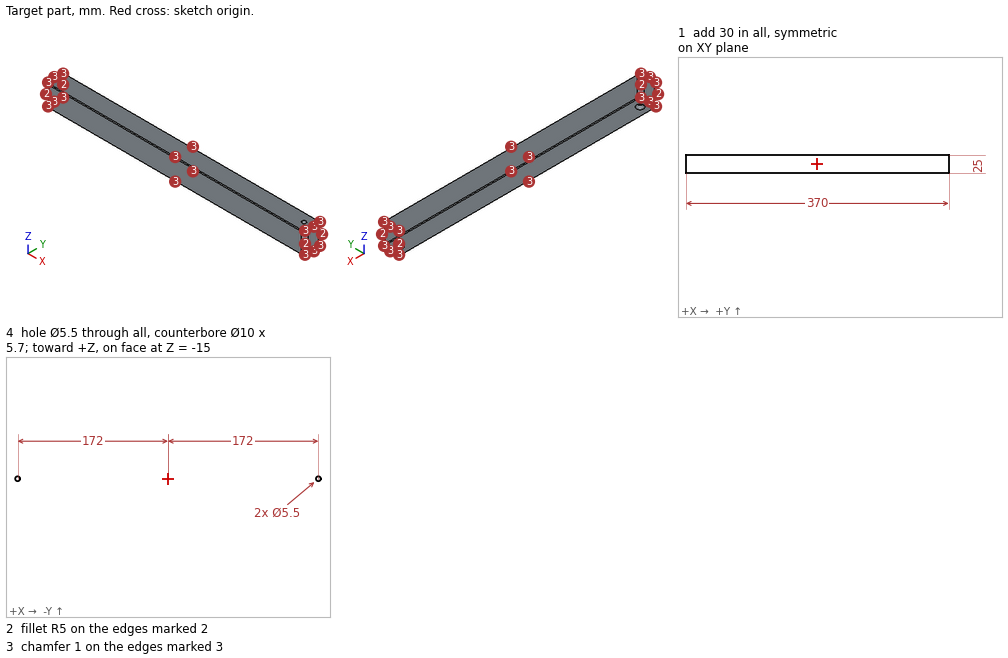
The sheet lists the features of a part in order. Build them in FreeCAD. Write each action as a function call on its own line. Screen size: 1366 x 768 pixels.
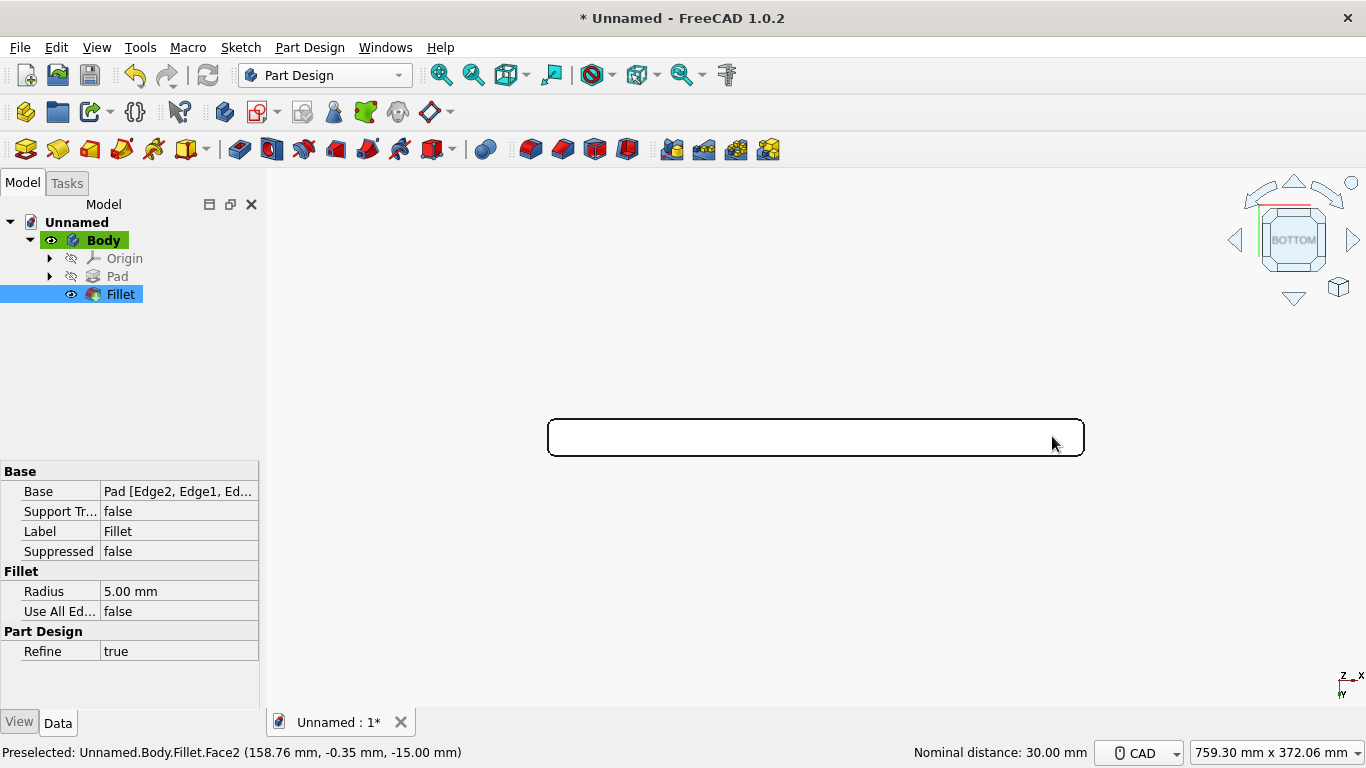
click(564, 150)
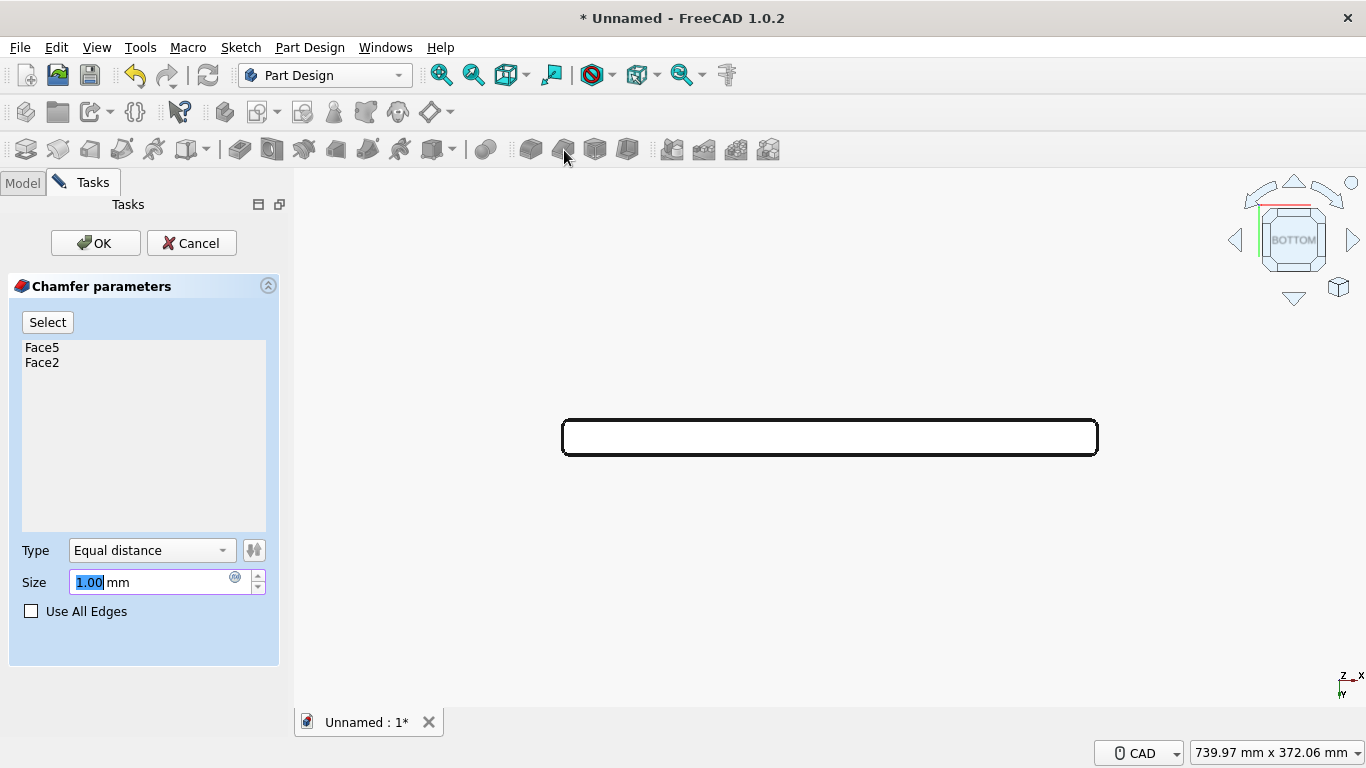
text(1)
key(Tab)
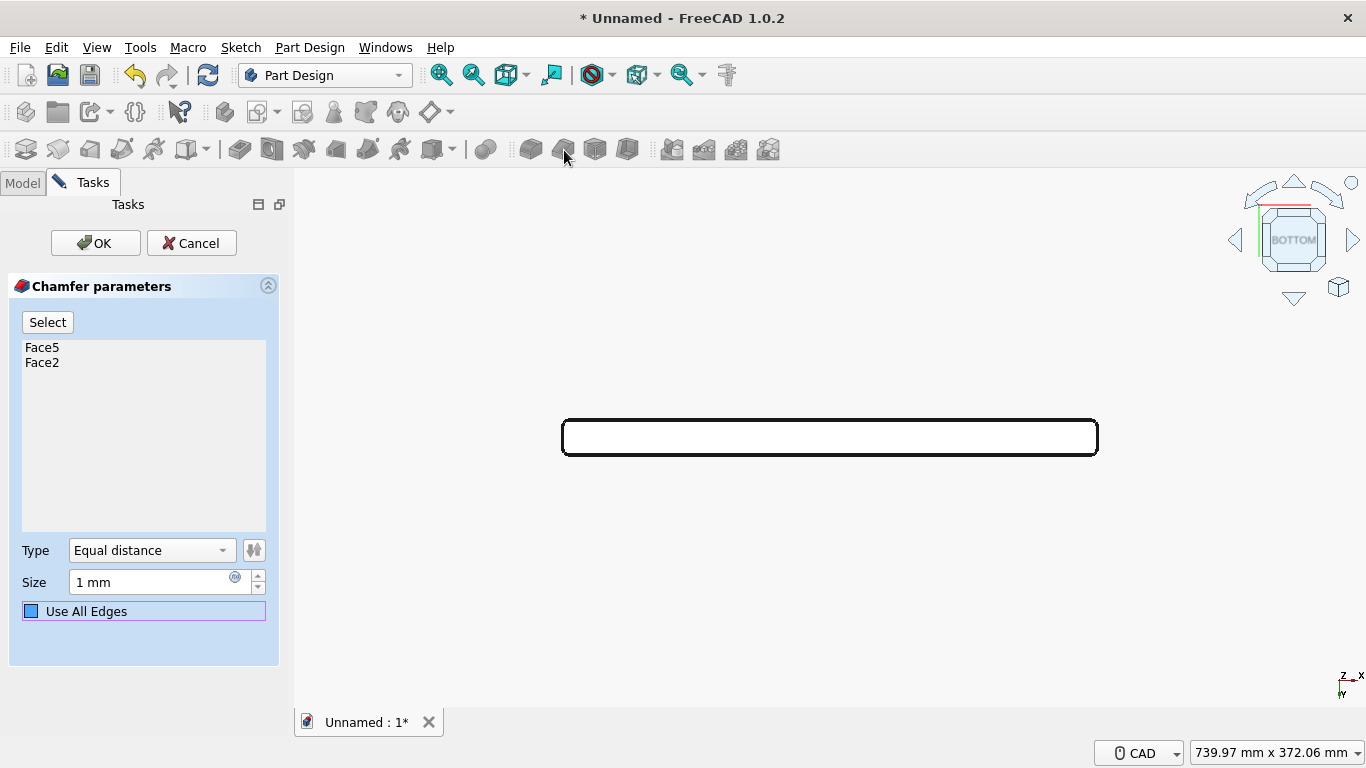
click(96, 243)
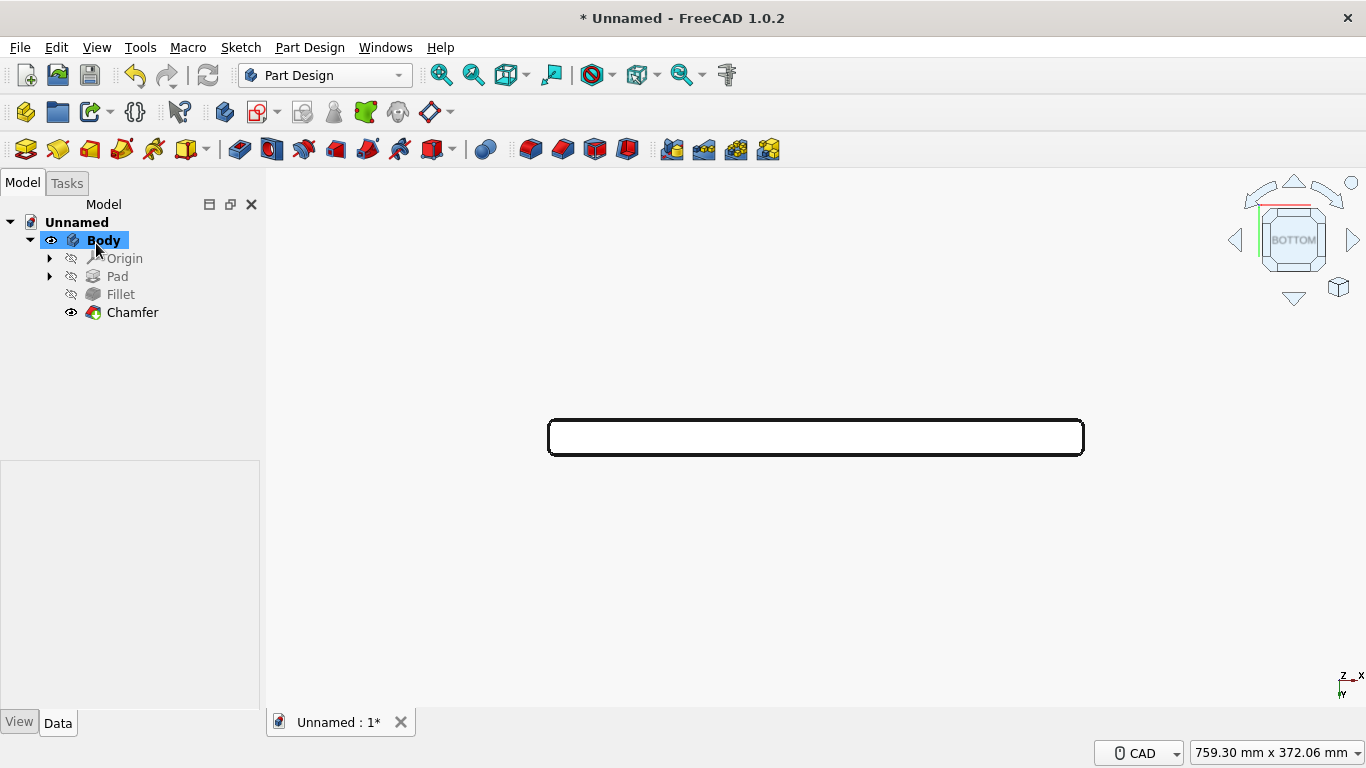
click(1044, 436)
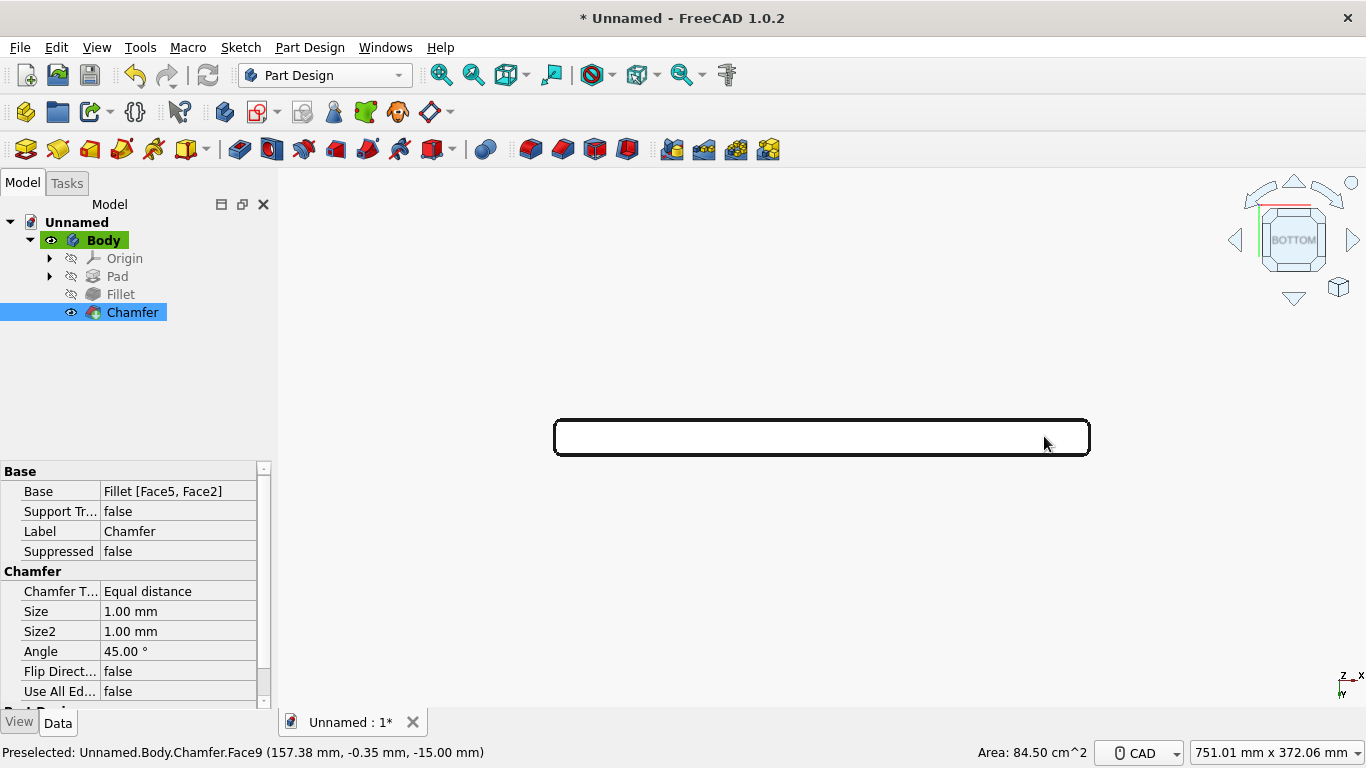
click(258, 112)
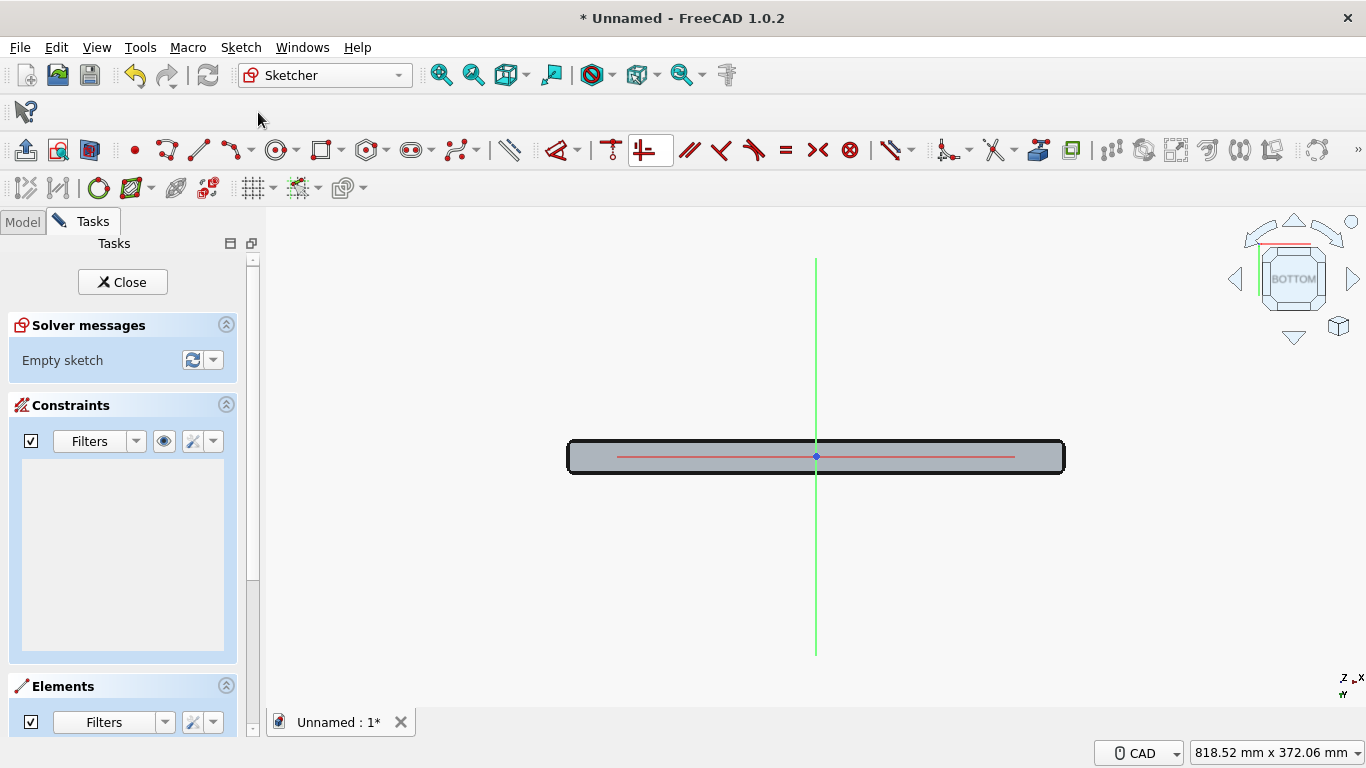
scroll(955, 457, up, 2)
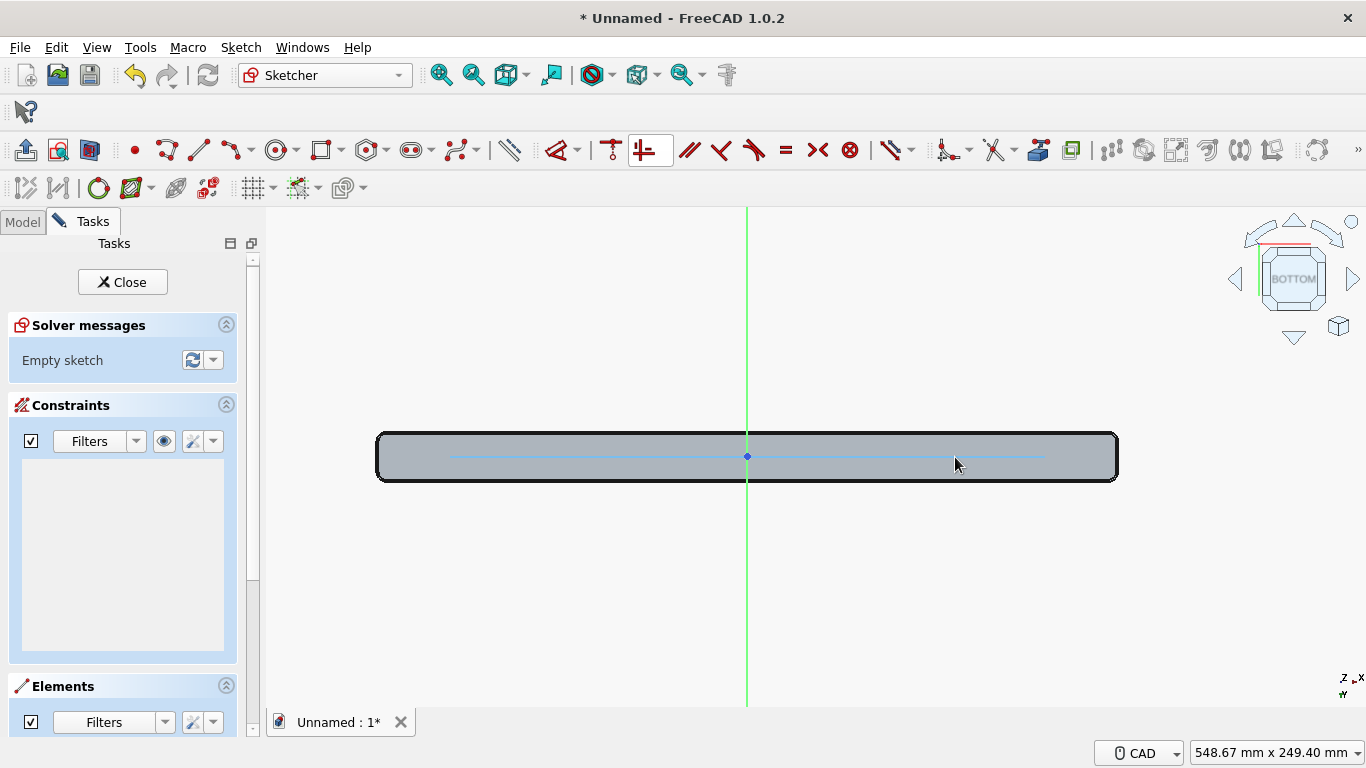
key(g)
key(c)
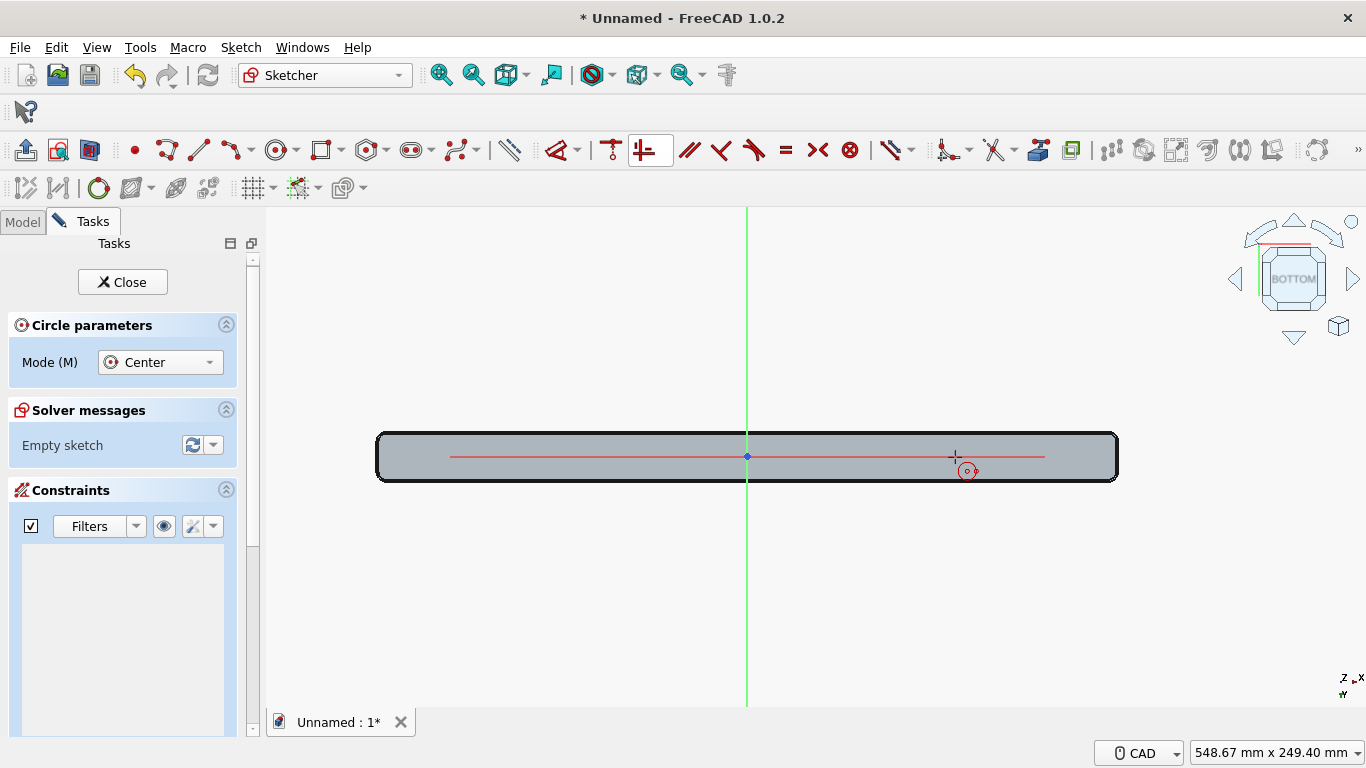
scroll(1092, 457, up, 8)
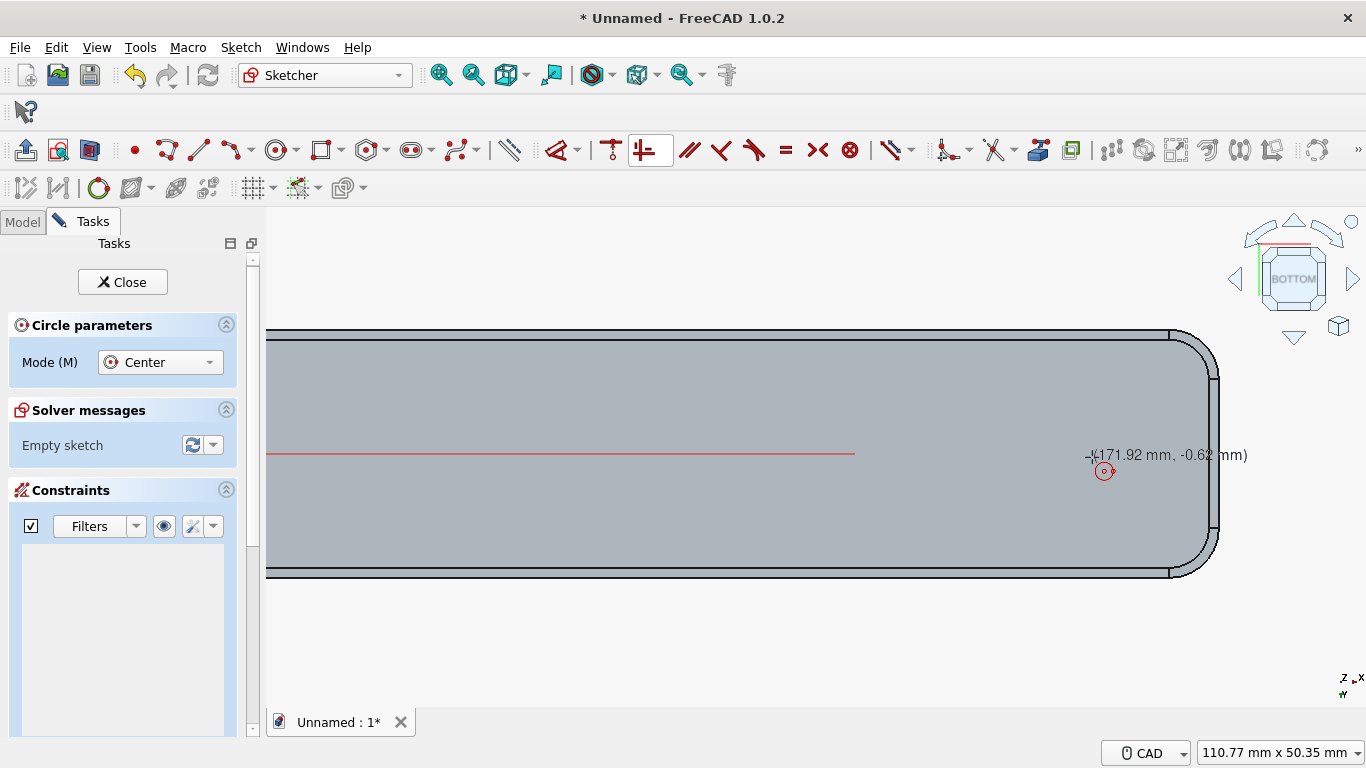
scroll(1093, 458, down, 8)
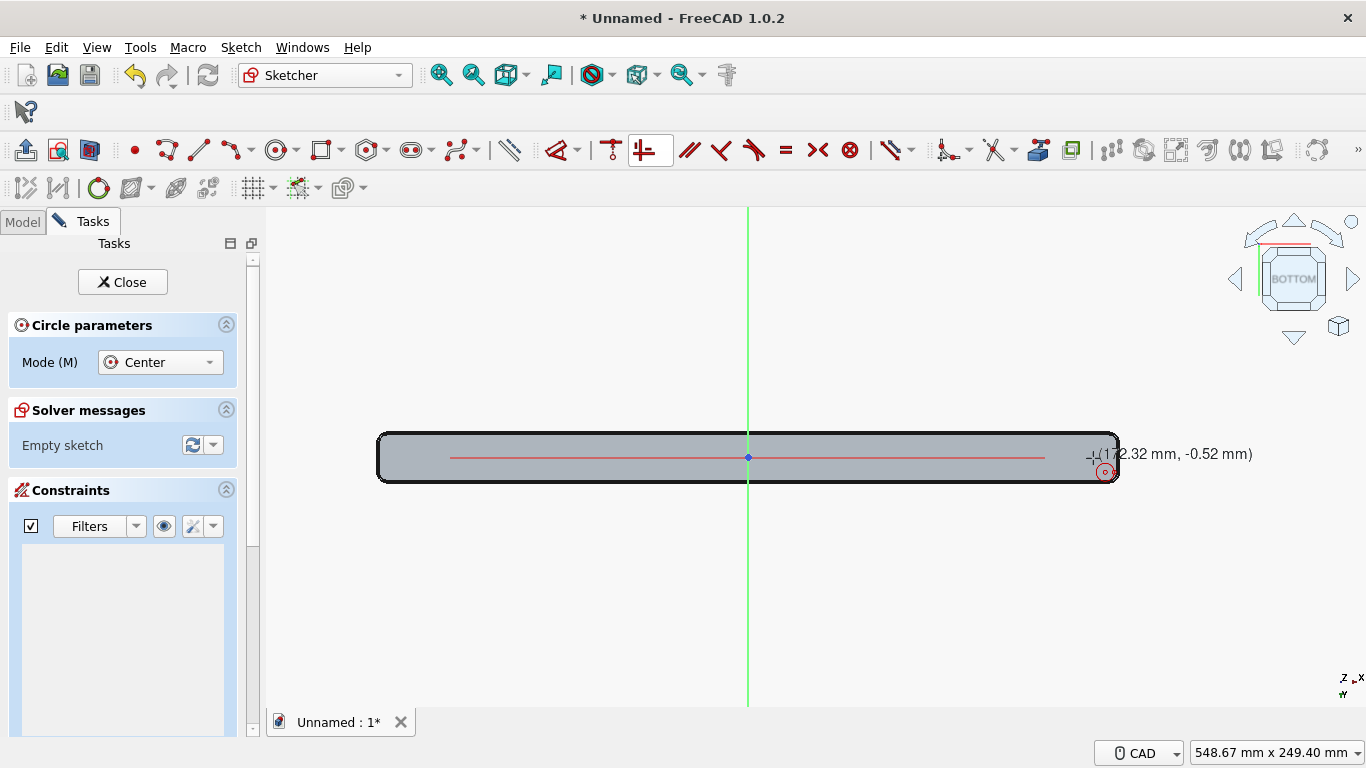
click(1093, 458)